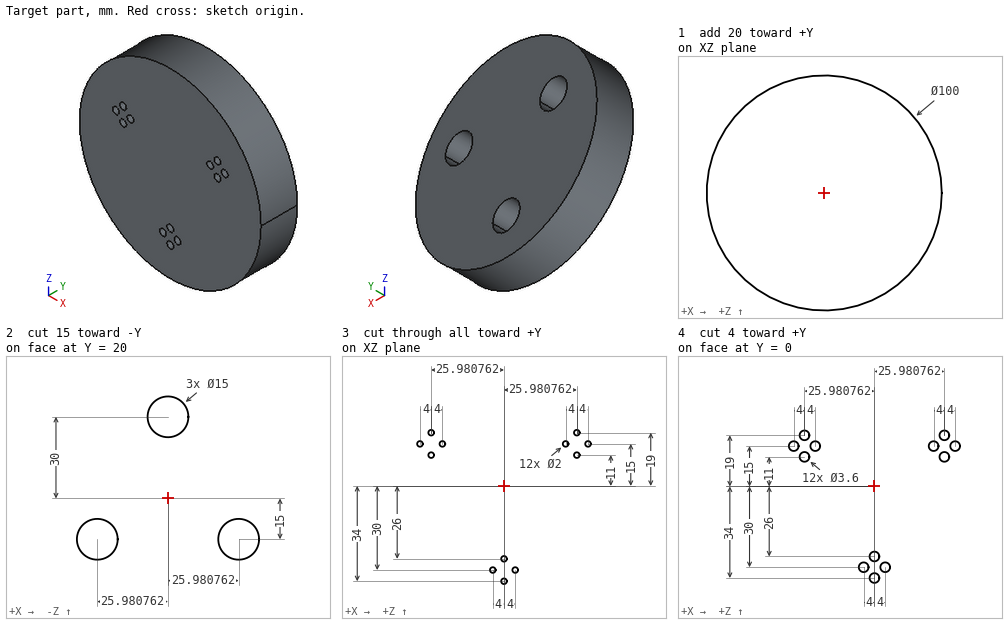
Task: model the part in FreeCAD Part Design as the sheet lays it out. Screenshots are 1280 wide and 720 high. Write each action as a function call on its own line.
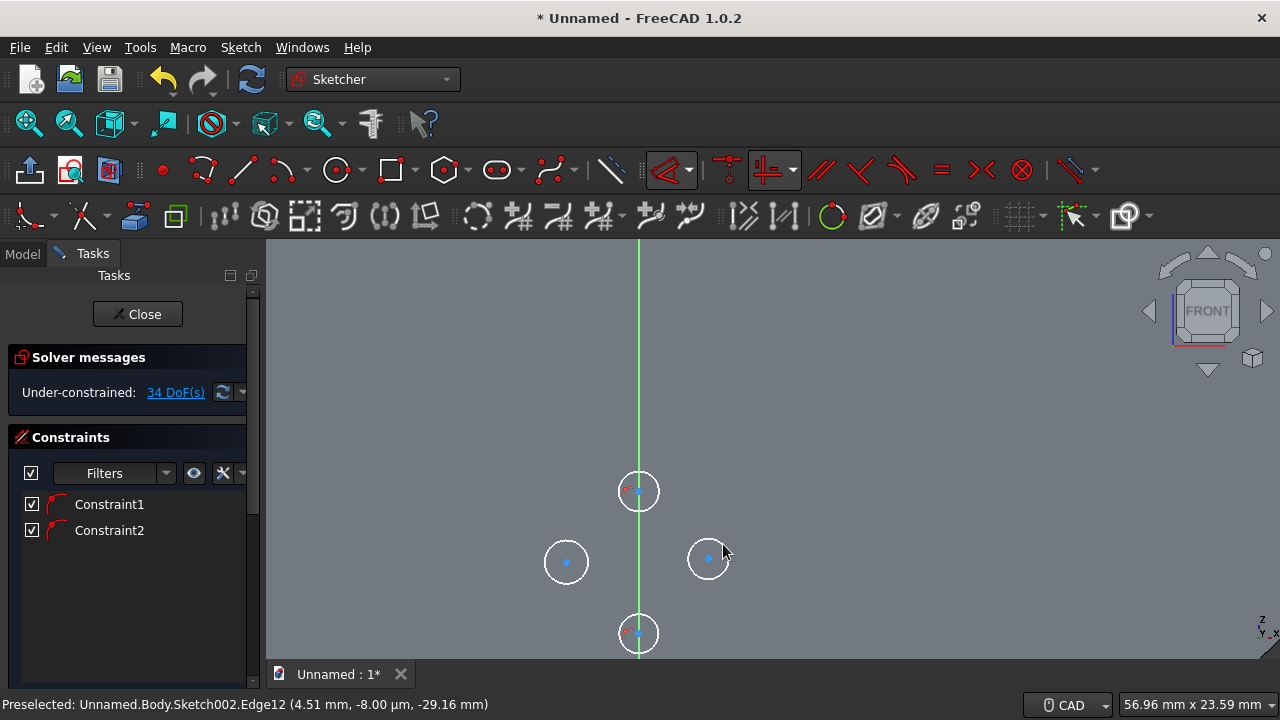
scroll(726, 545, down, 7)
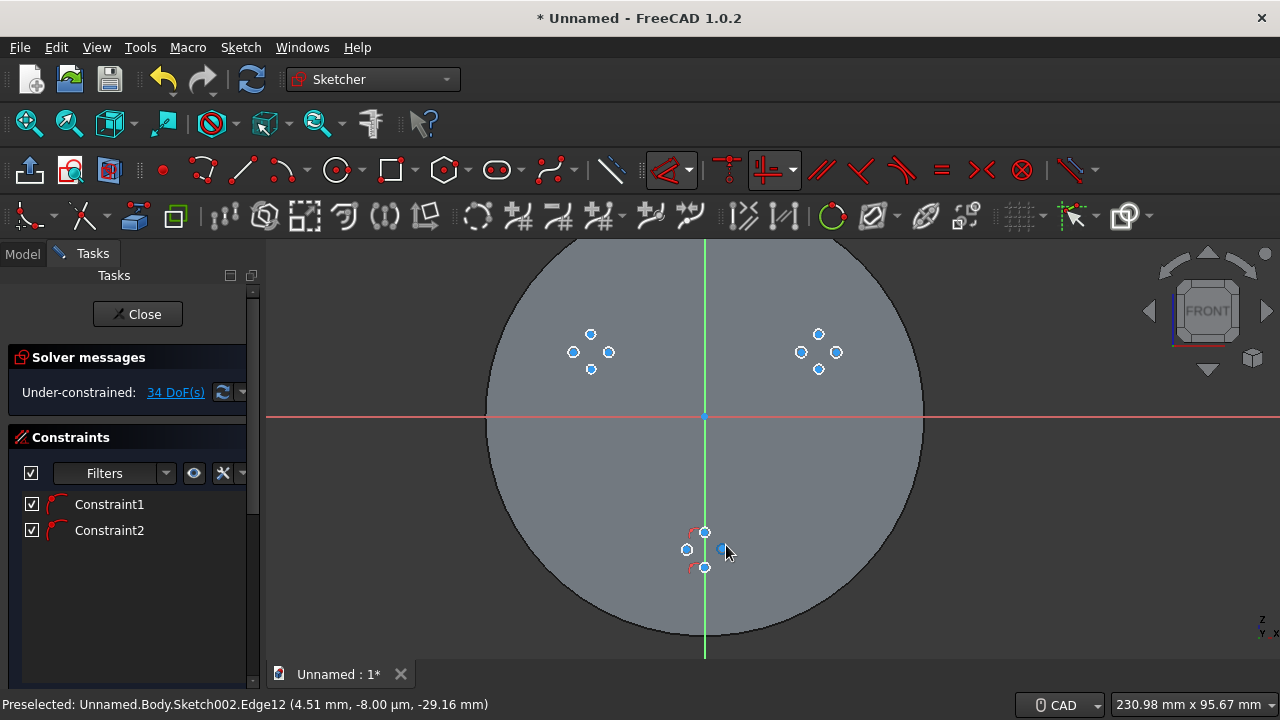
scroll(822, 331, up, 6)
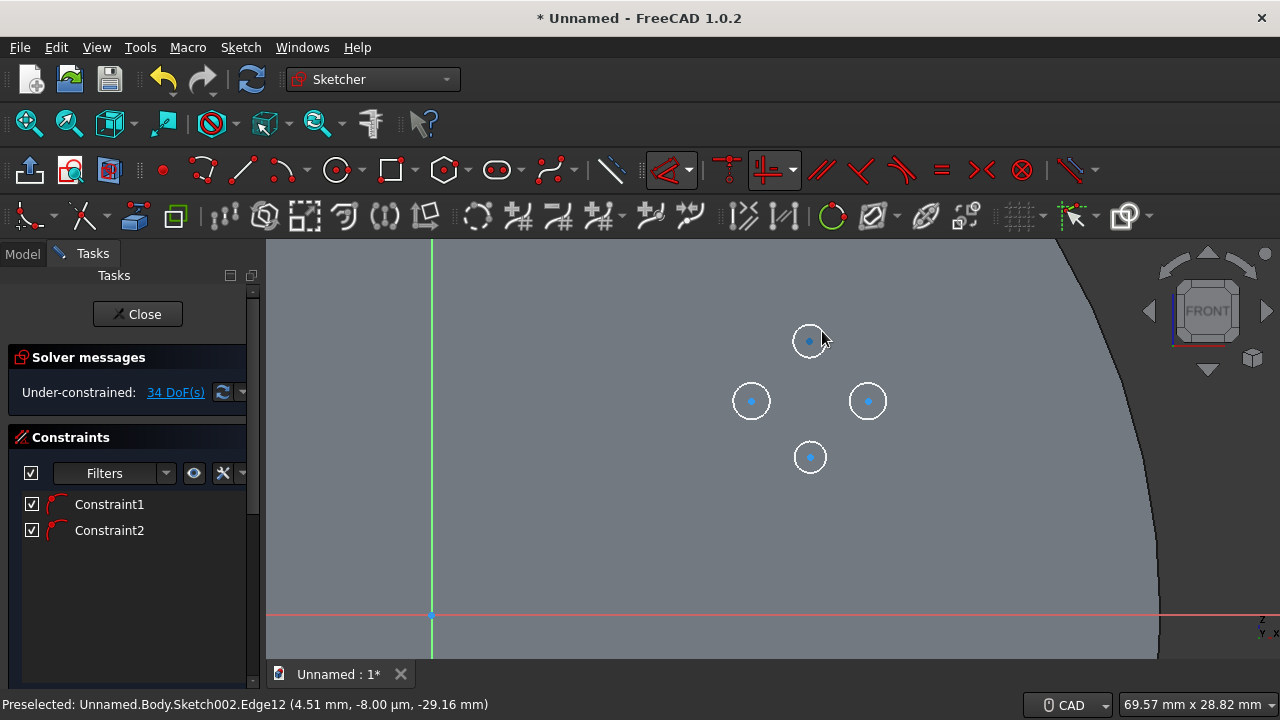
click(821, 329)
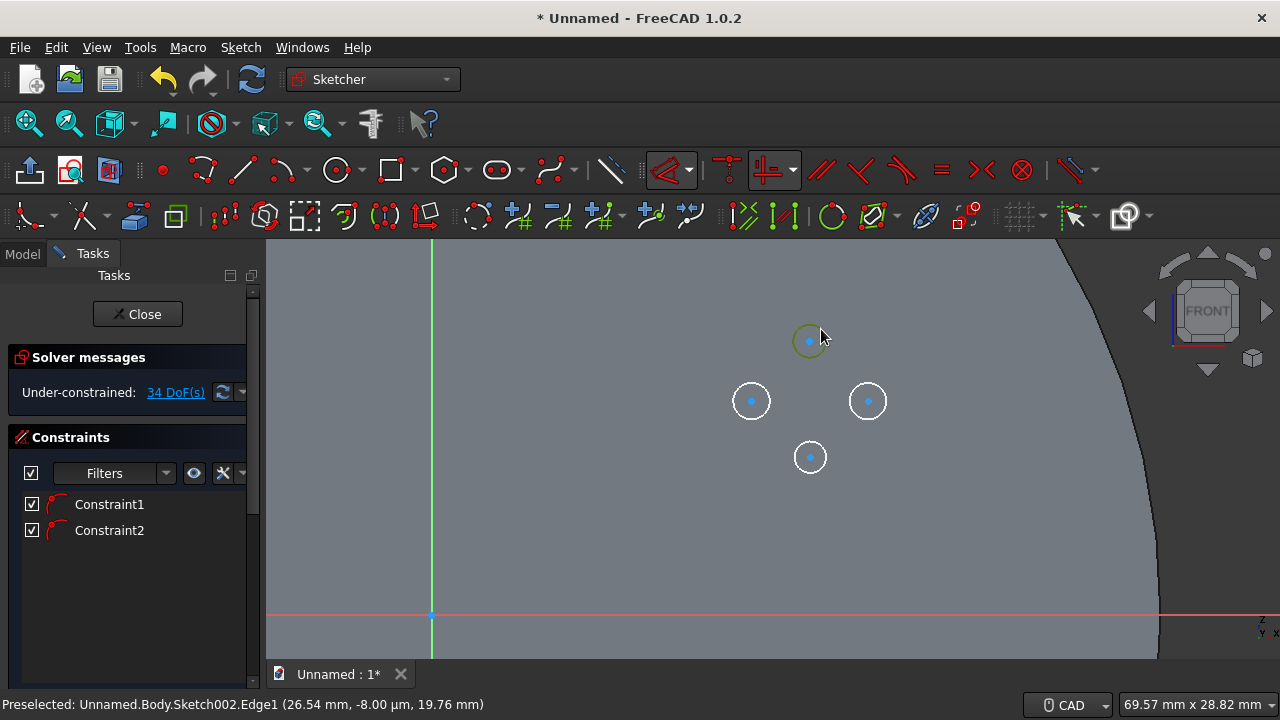
click(881, 388)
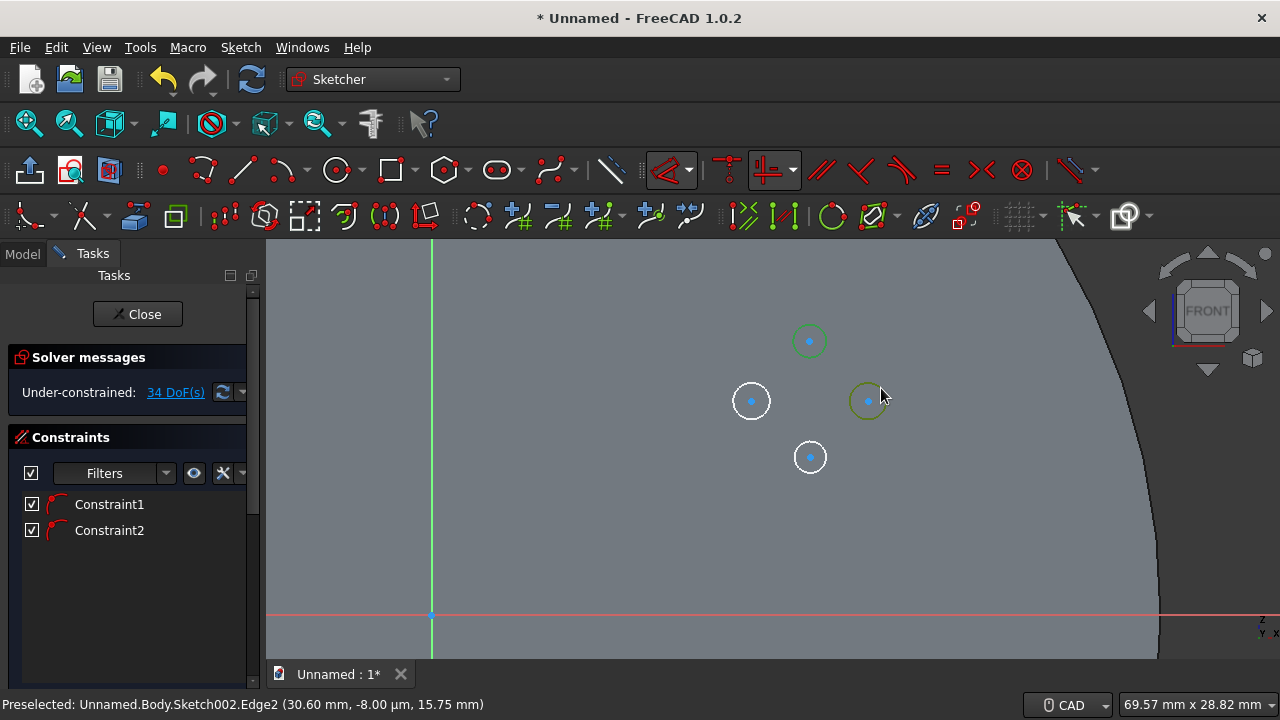
click(764, 388)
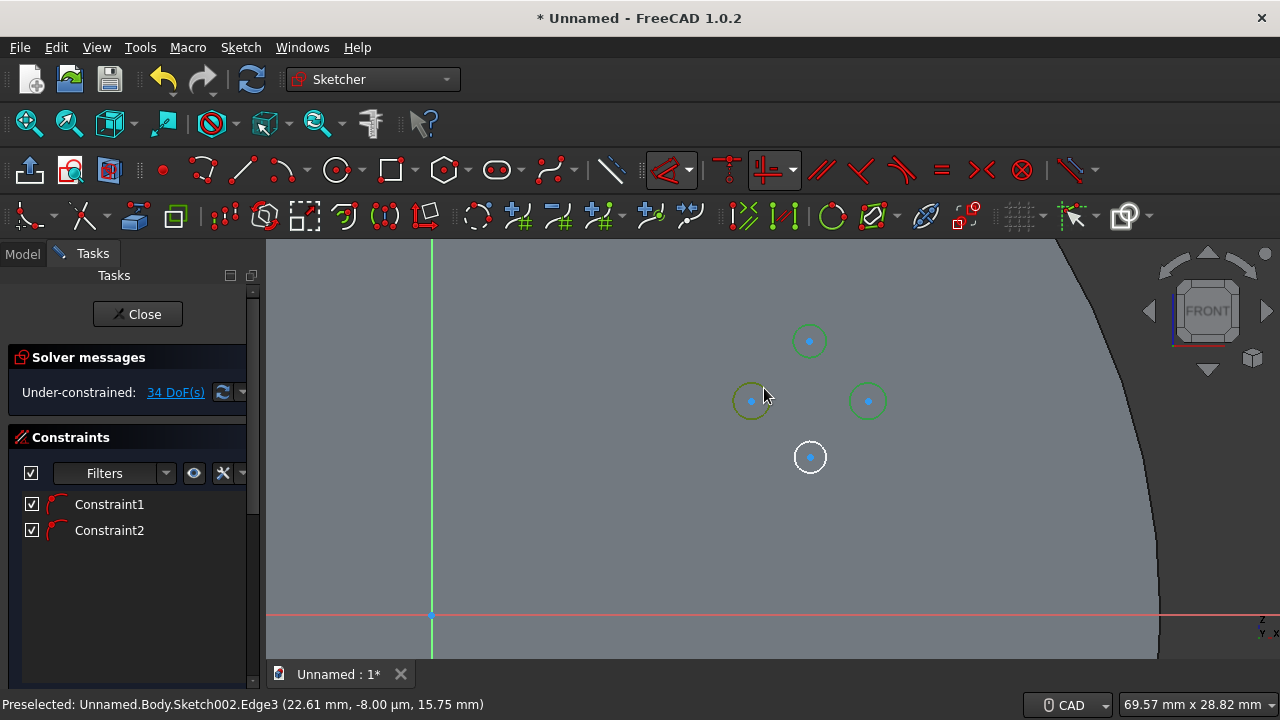
click(821, 446)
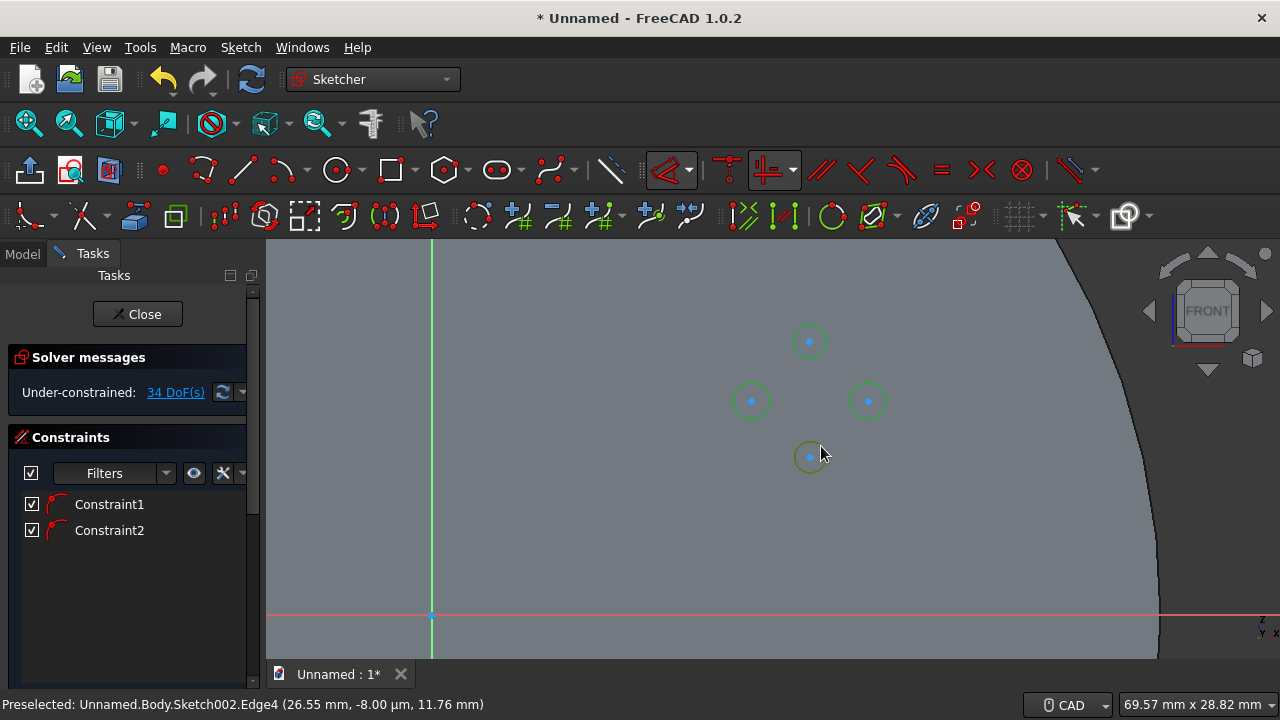
scroll(822, 330, down, 6)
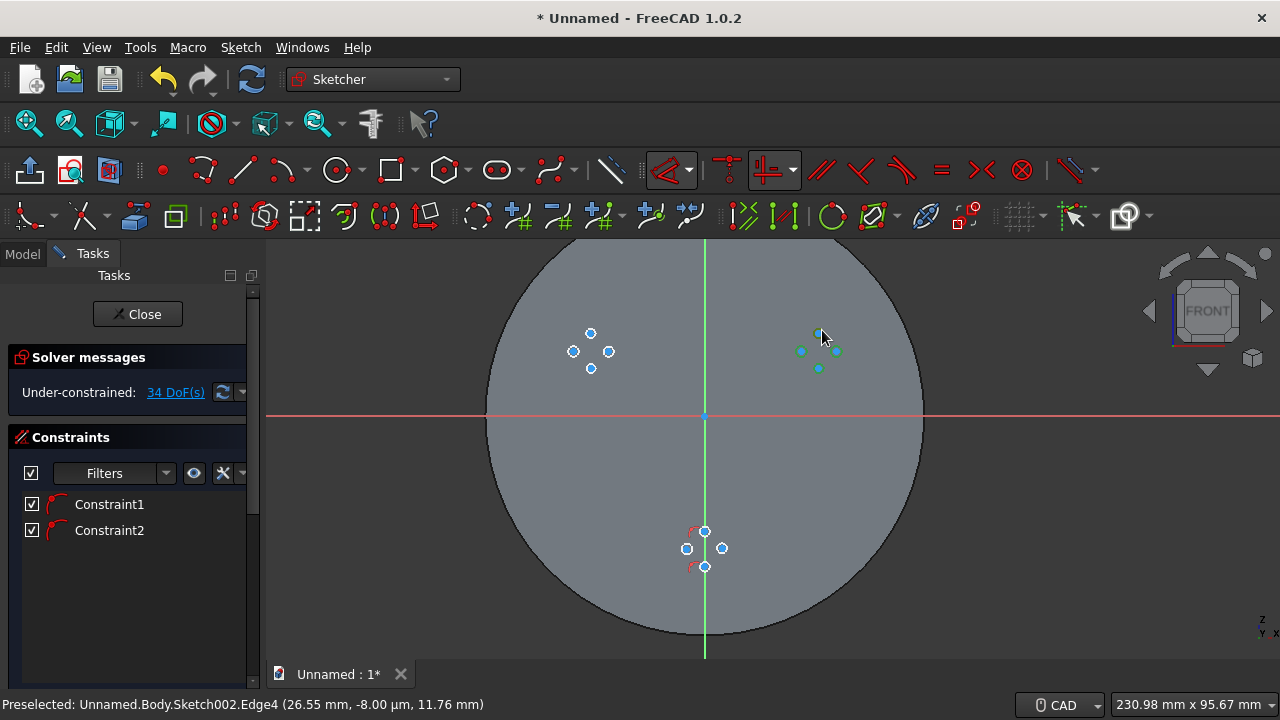
scroll(594, 330, up, 6)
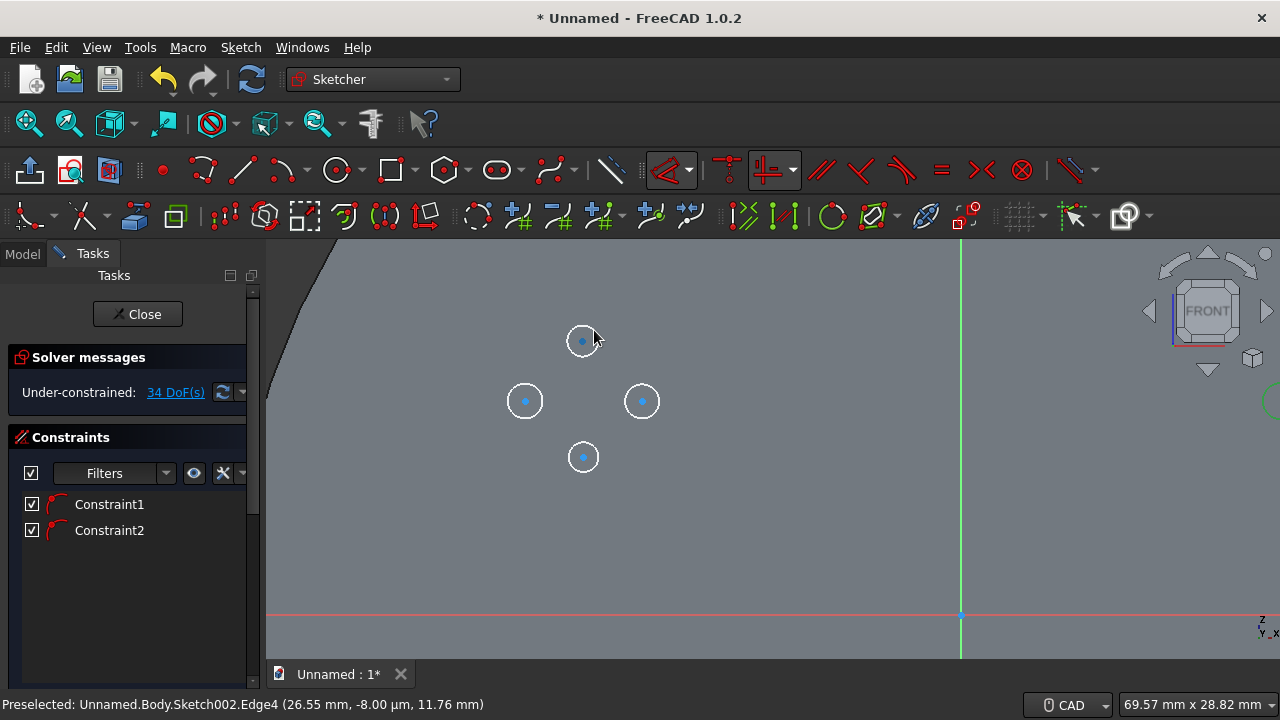
click(594, 330)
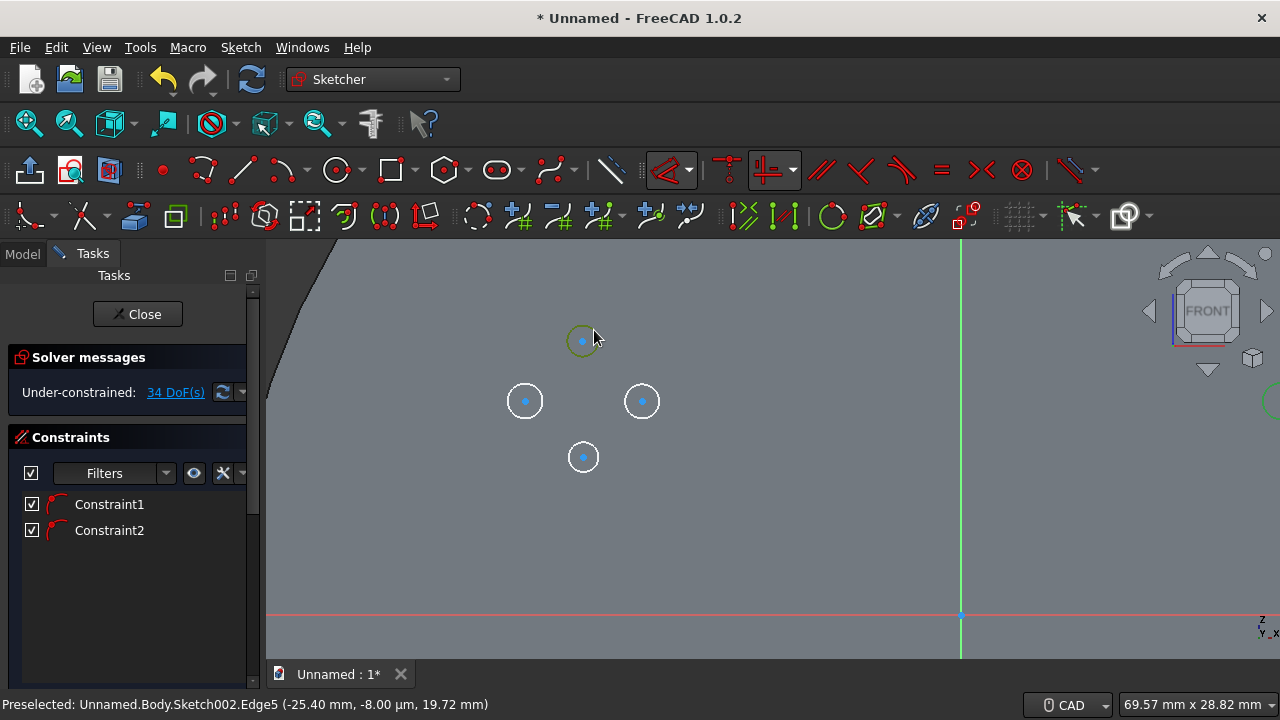
click(537, 389)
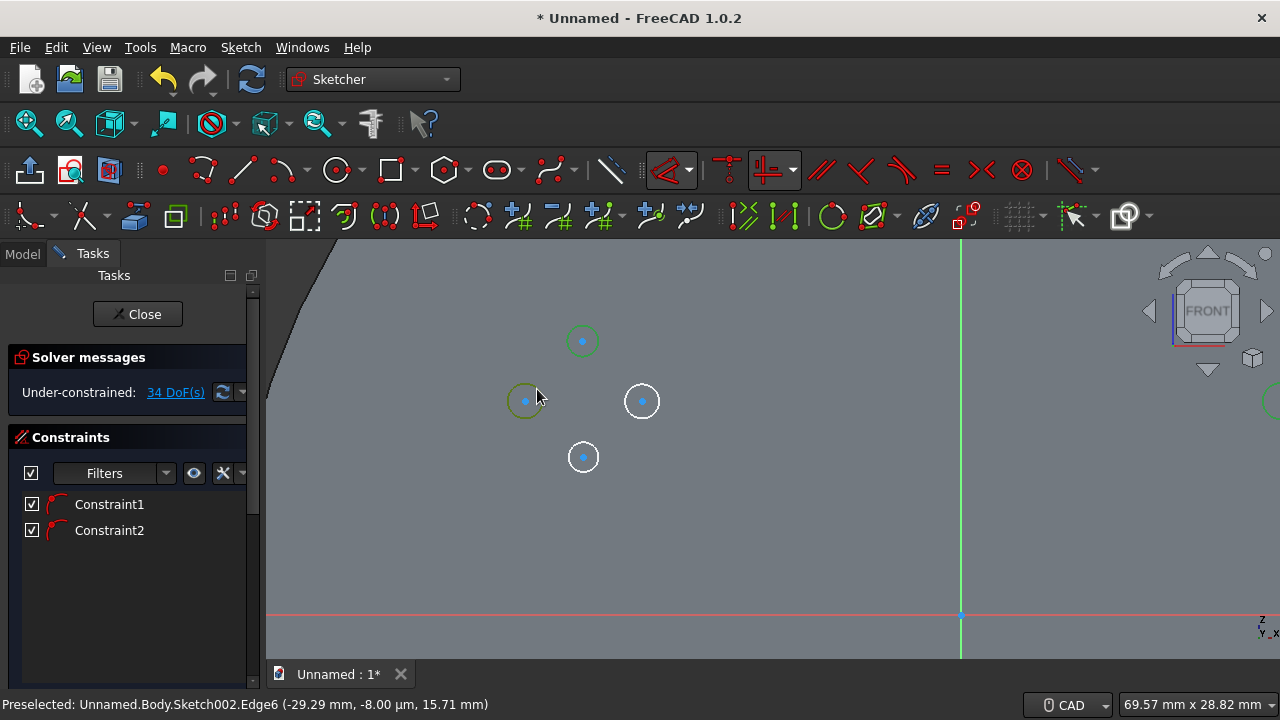
click(594, 447)